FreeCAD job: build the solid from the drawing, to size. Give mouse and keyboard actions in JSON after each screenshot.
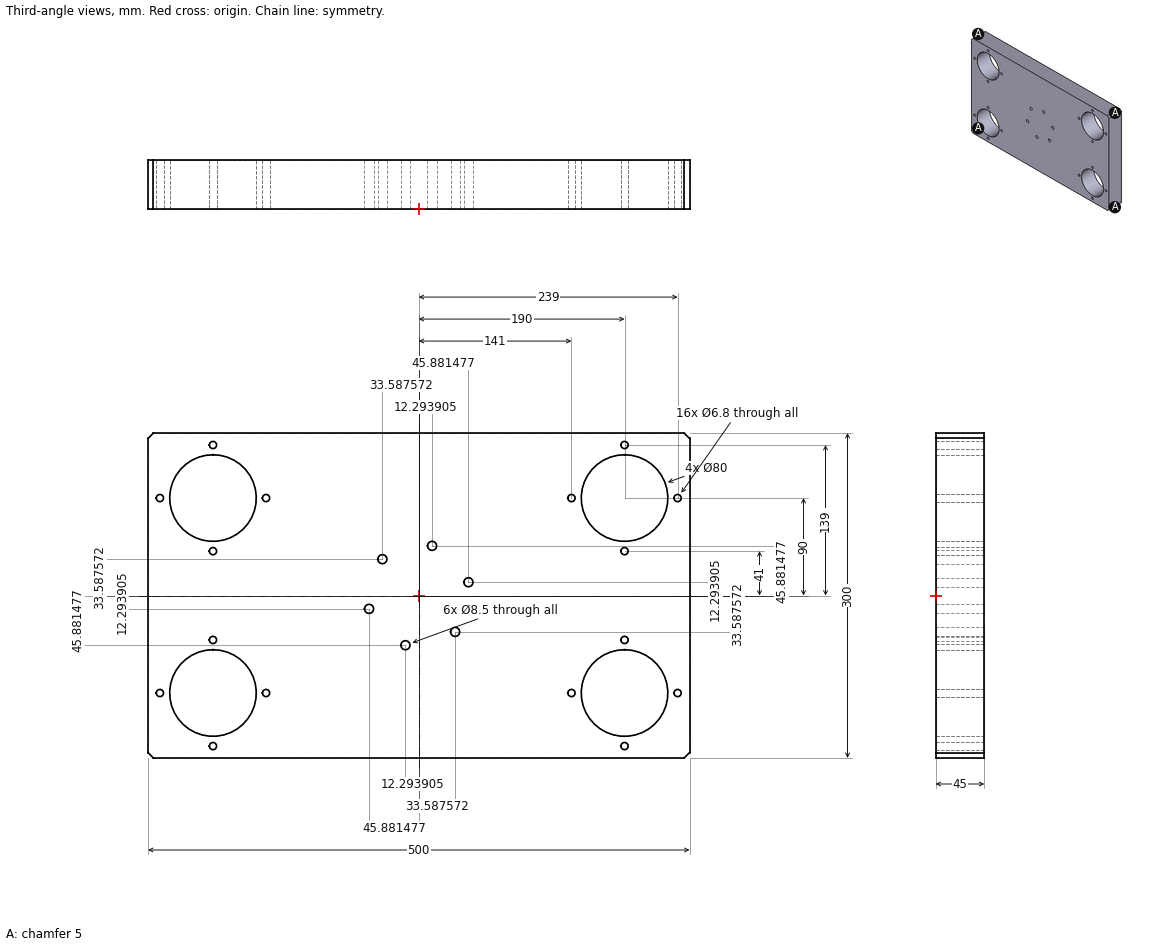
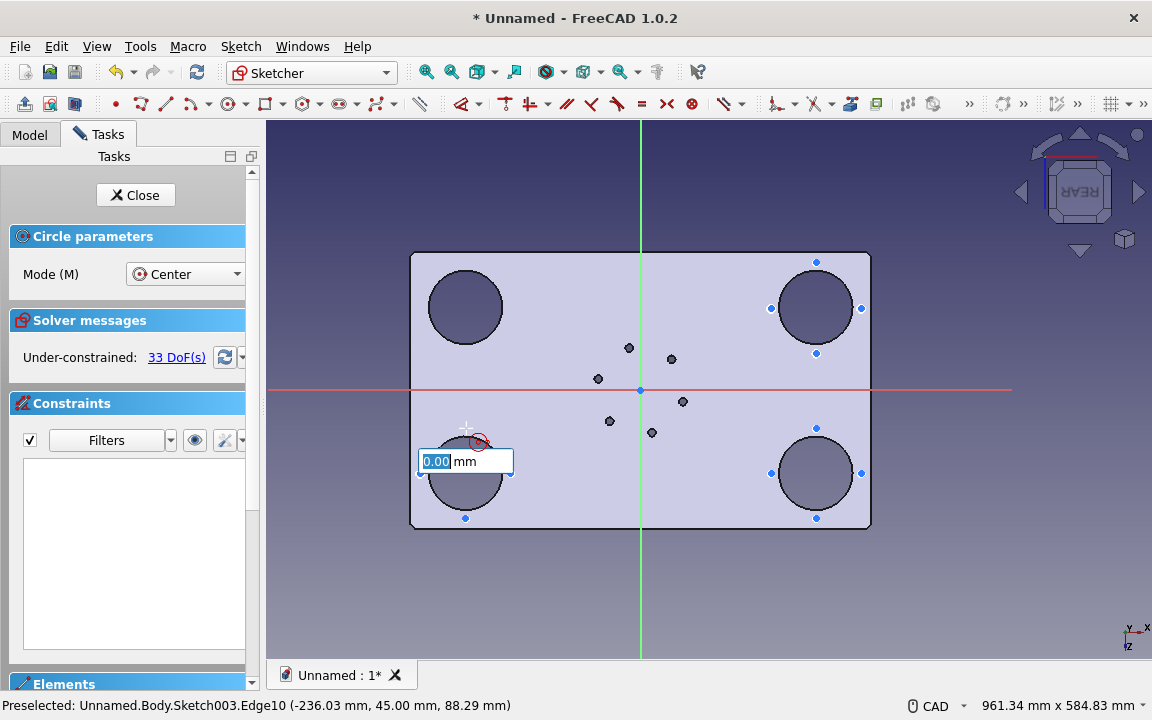
{"action": "scroll", "coordinate": [468, 426], "scroll_direction": "up", "scroll_amount": 9}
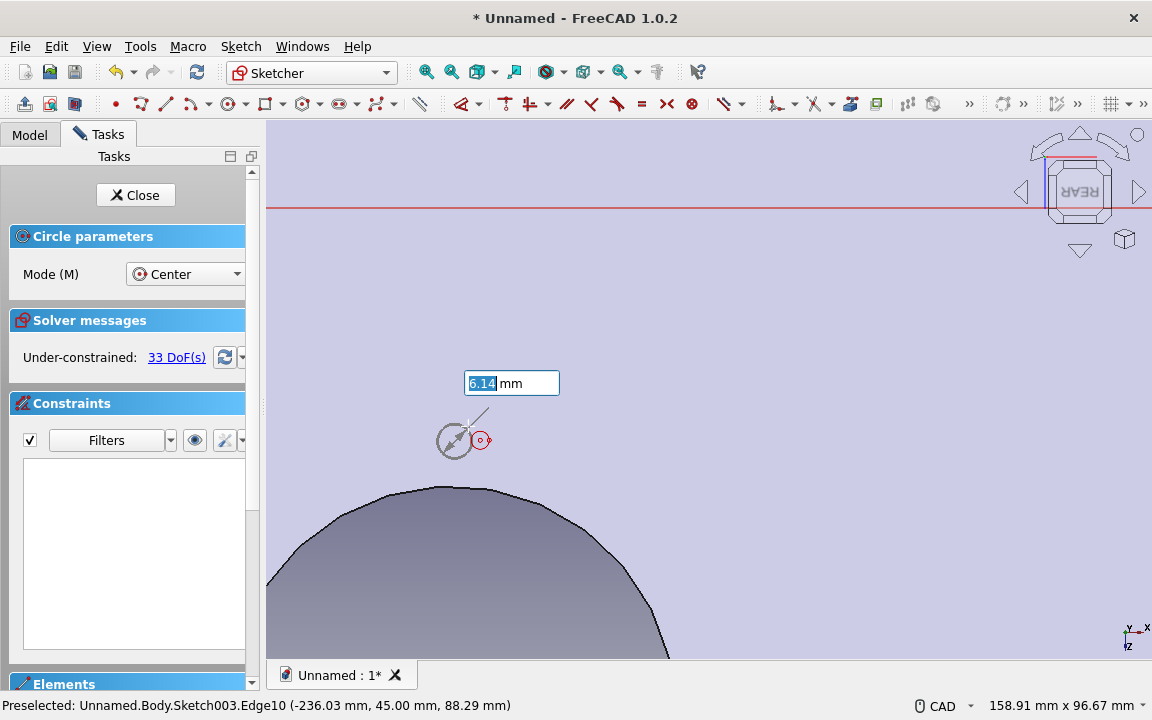
{"action": "left_click", "coordinate": [465, 423]}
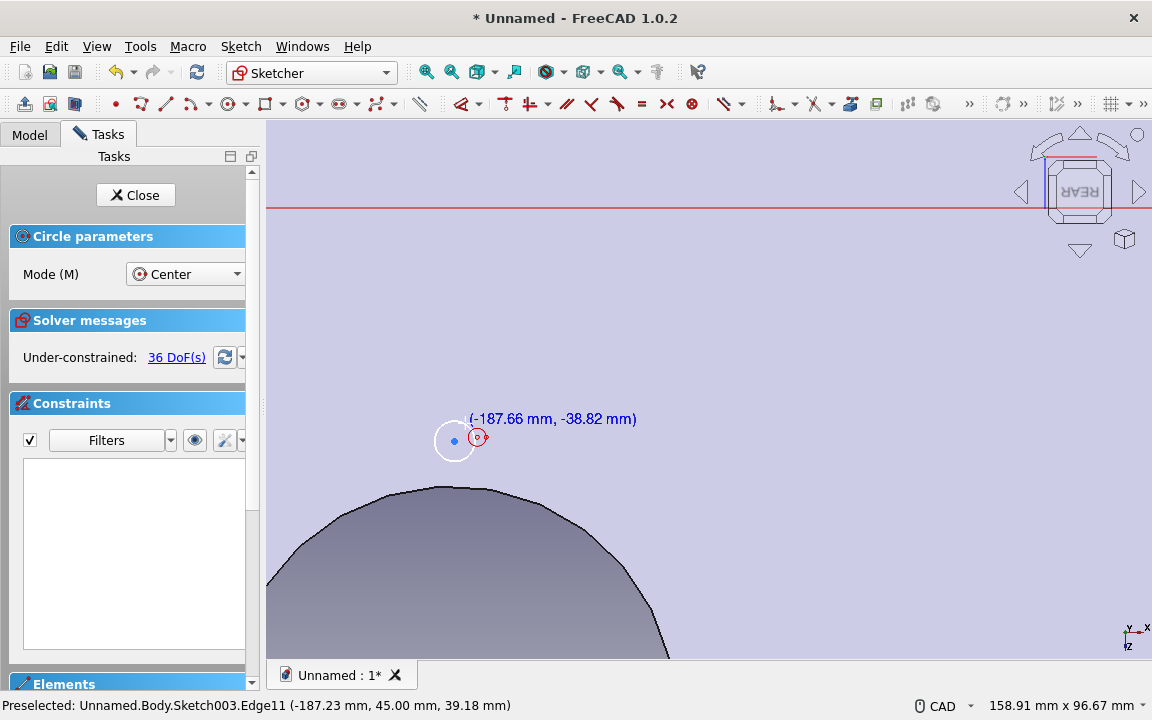
{"action": "scroll", "coordinate": [468, 426], "scroll_direction": "down", "scroll_amount": 9}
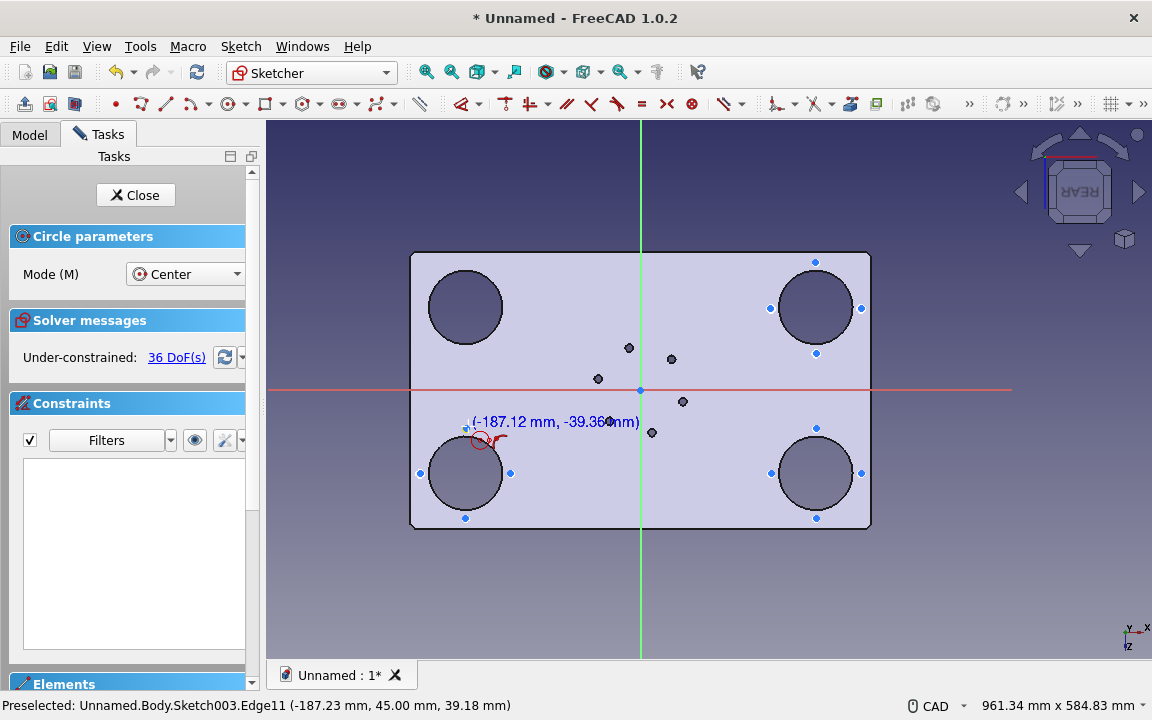
{"action": "scroll", "coordinate": [511, 307], "scroll_direction": "up", "scroll_amount": 10}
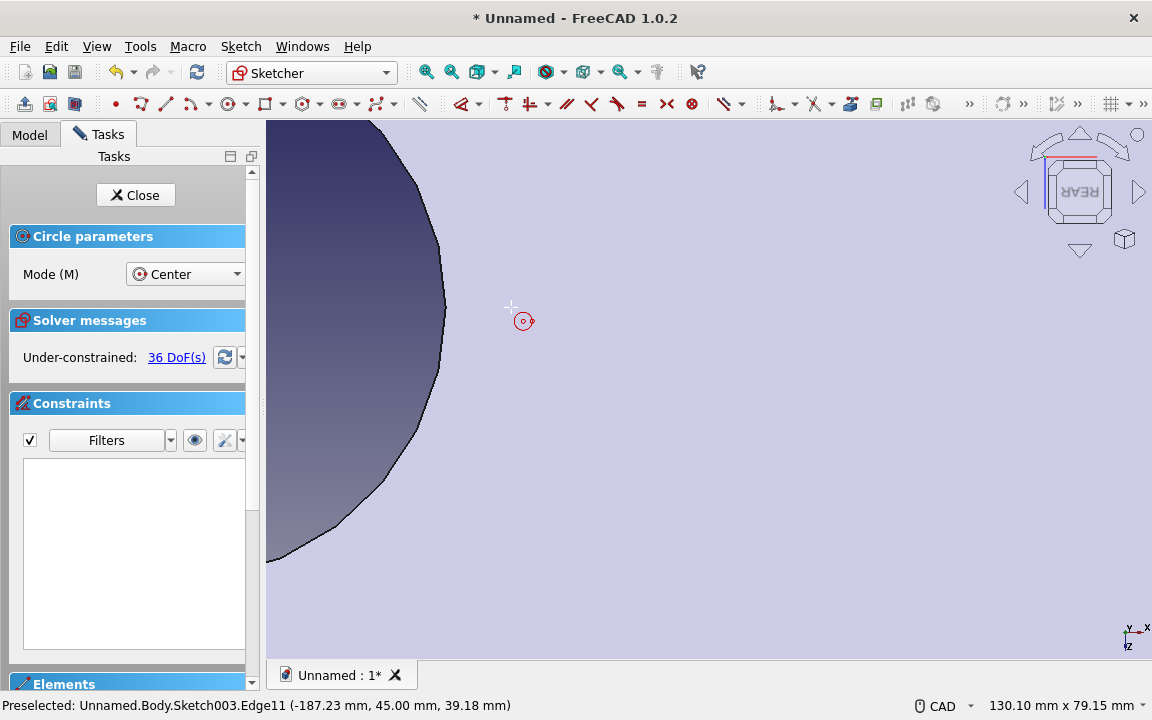
{"action": "scroll", "coordinate": [511, 306], "scroll_direction": "down", "scroll_amount": 10}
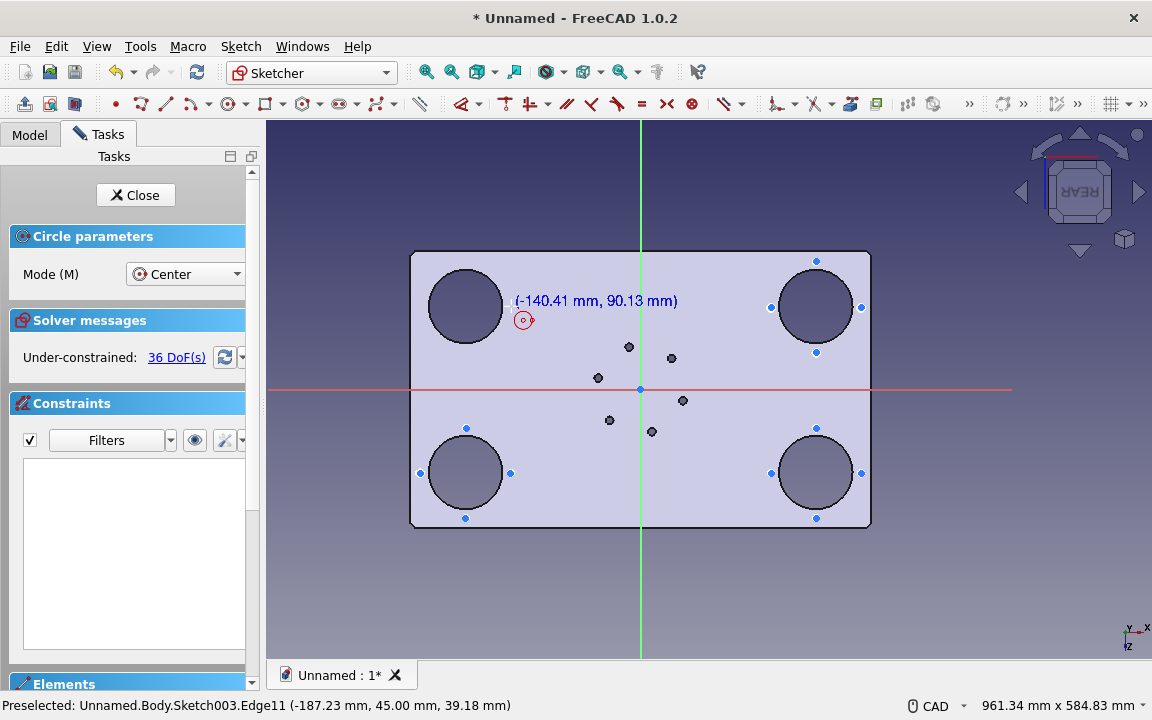
{"action": "left_click", "coordinate": [511, 307]}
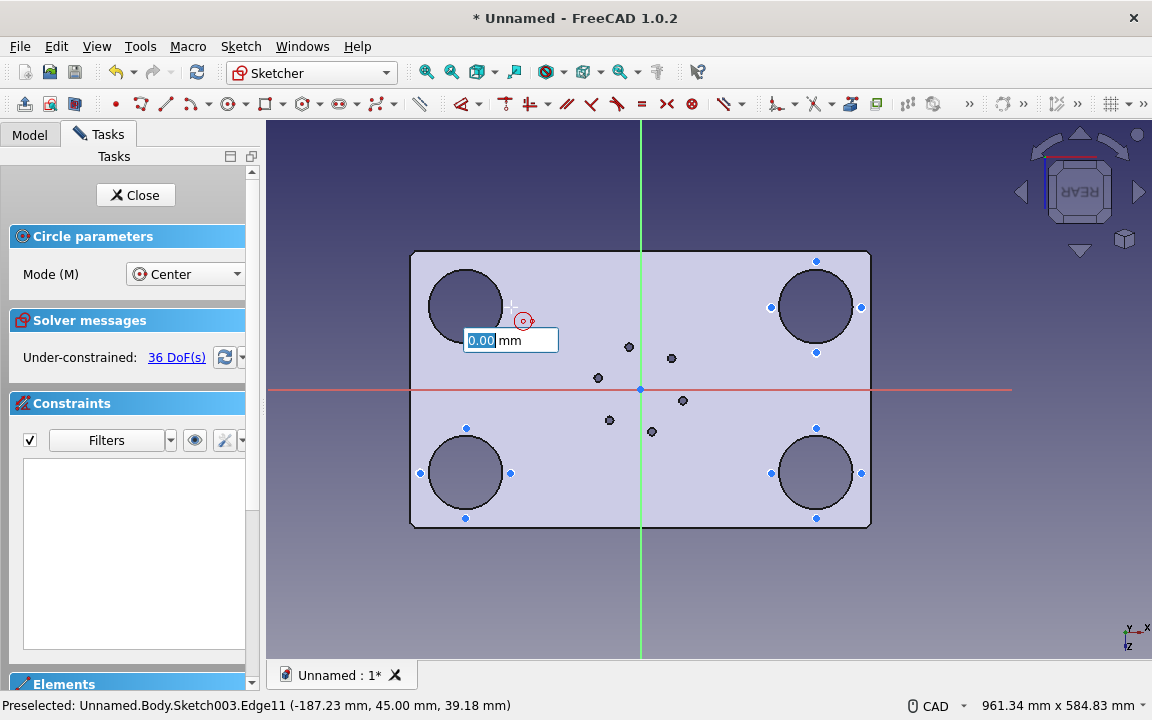
{"action": "scroll", "coordinate": [513, 304], "scroll_direction": "up", "scroll_amount": 9}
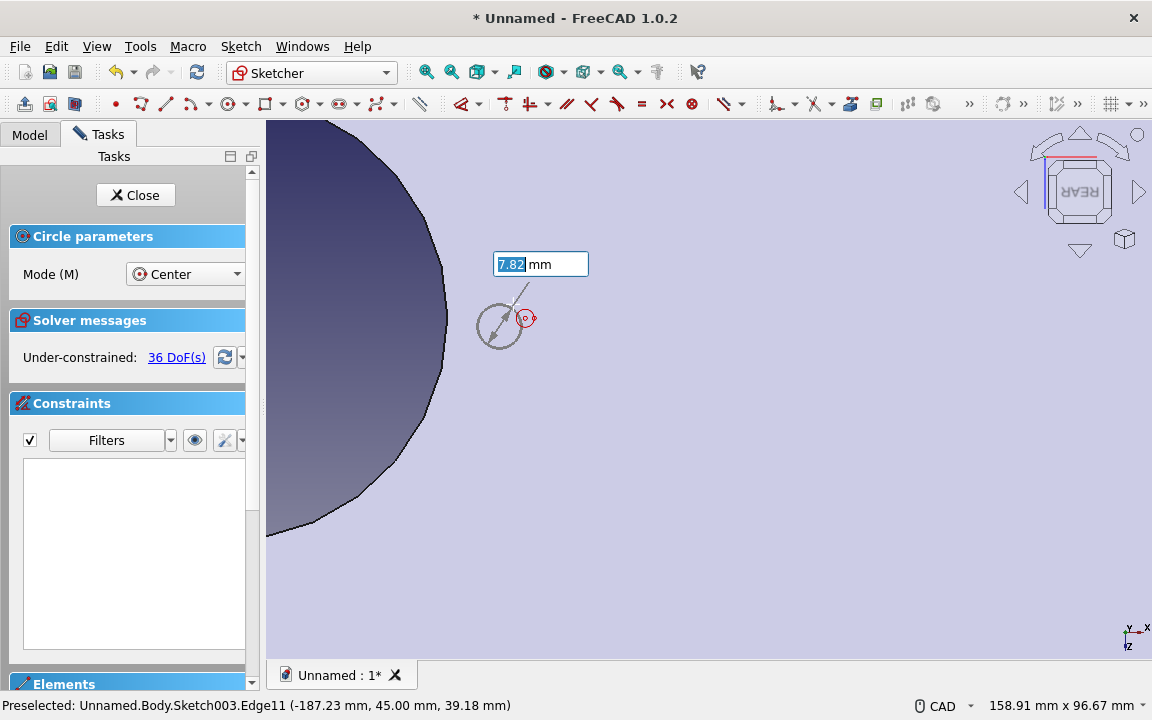
{"action": "left_click", "coordinate": [511, 304]}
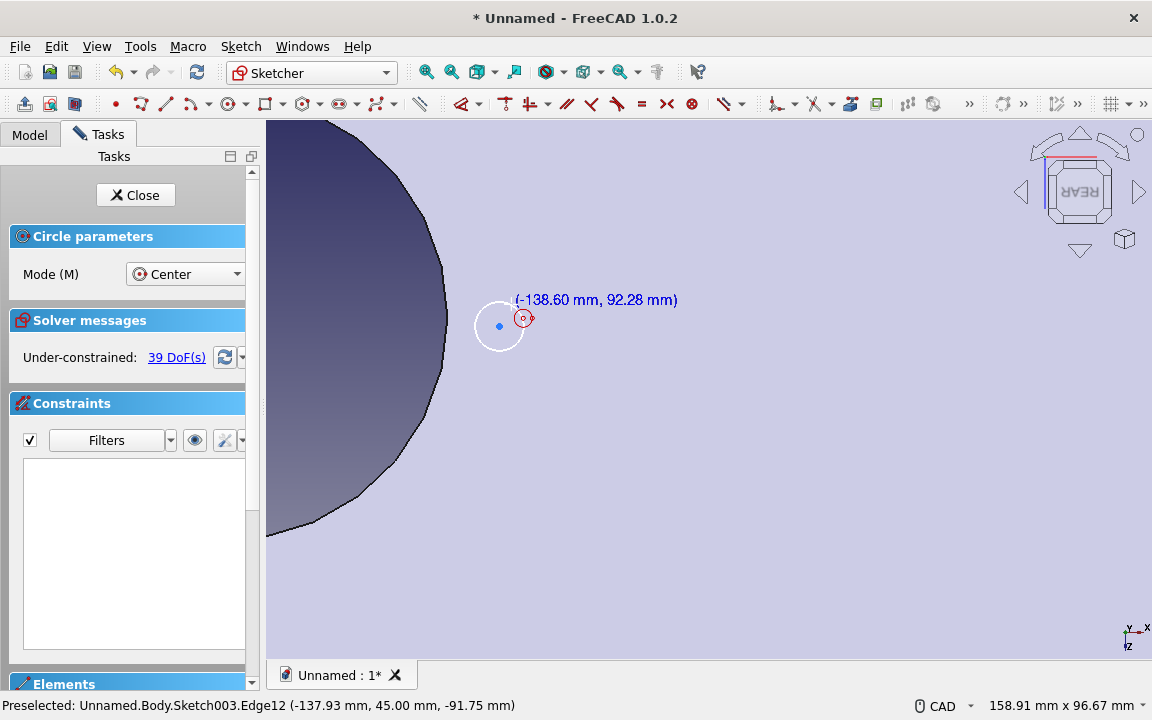
{"action": "scroll", "coordinate": [513, 304], "scroll_direction": "down", "scroll_amount": 9}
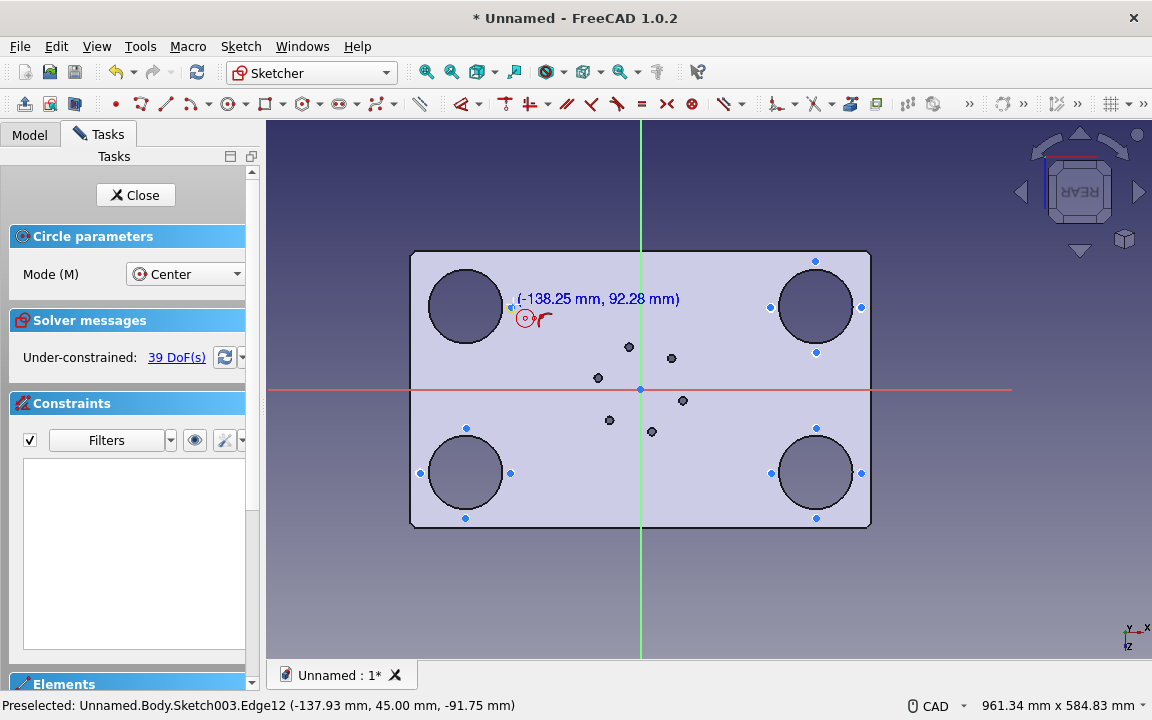
{"action": "scroll", "coordinate": [466, 352], "scroll_direction": "up", "scroll_amount": 10}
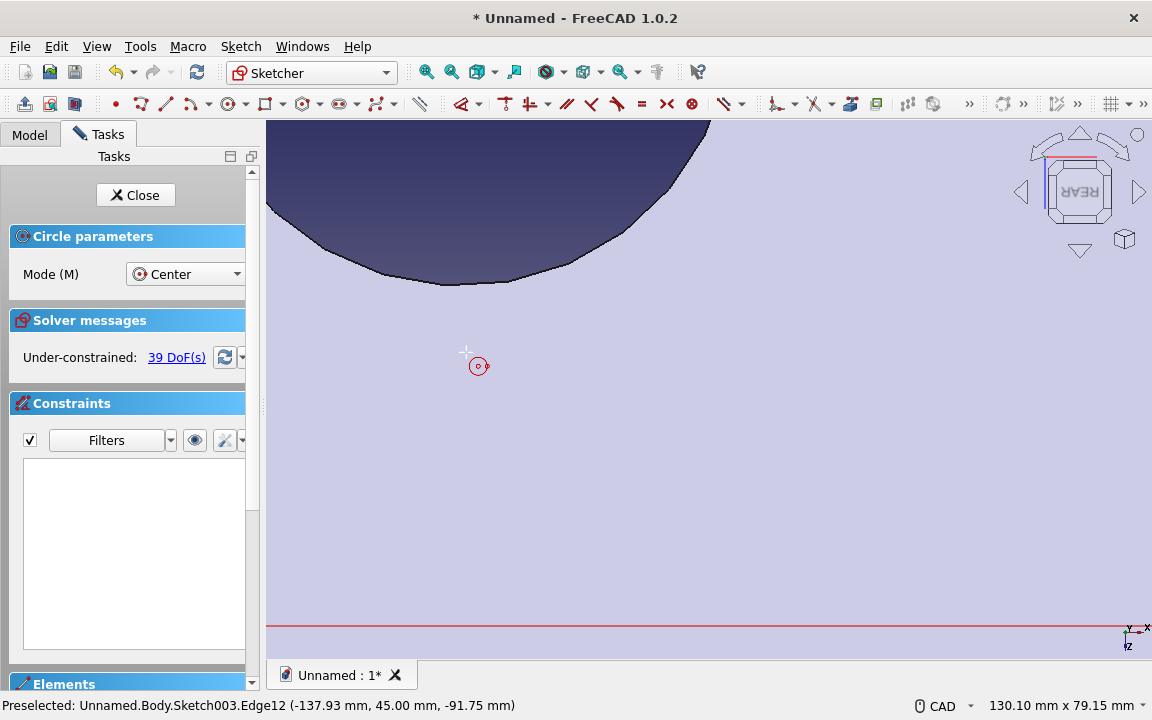
{"action": "scroll", "coordinate": [466, 352], "scroll_direction": "down", "scroll_amount": 10}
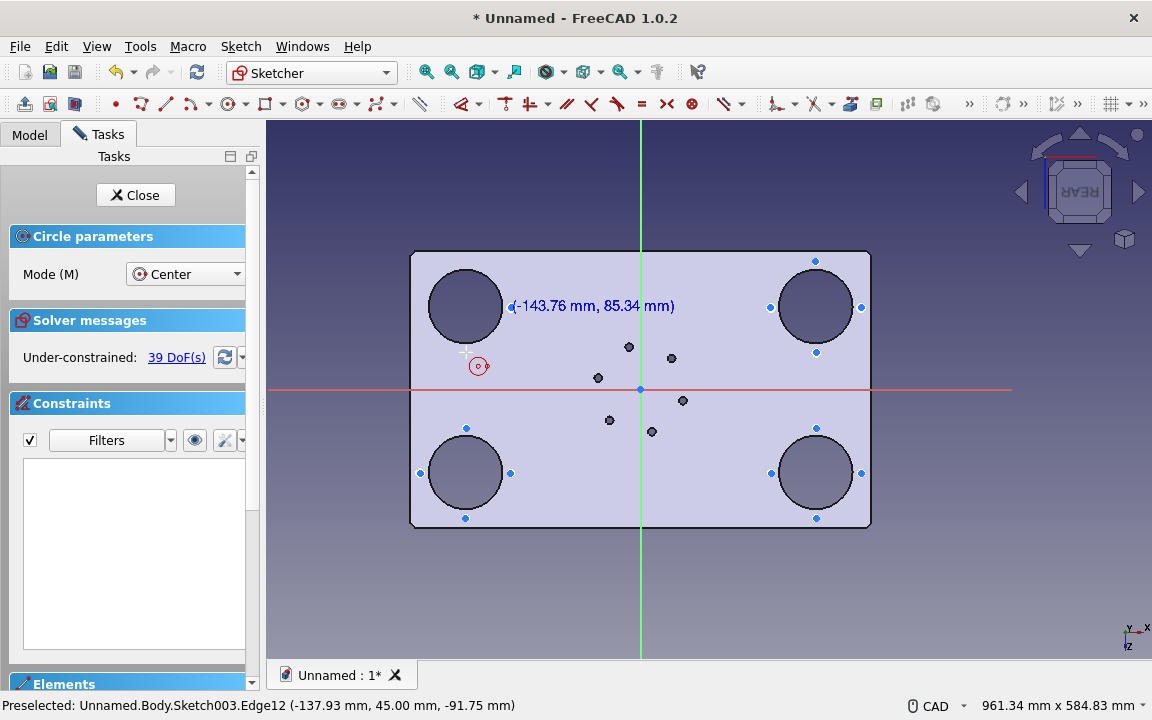
{"action": "left_click", "coordinate": [466, 352]}